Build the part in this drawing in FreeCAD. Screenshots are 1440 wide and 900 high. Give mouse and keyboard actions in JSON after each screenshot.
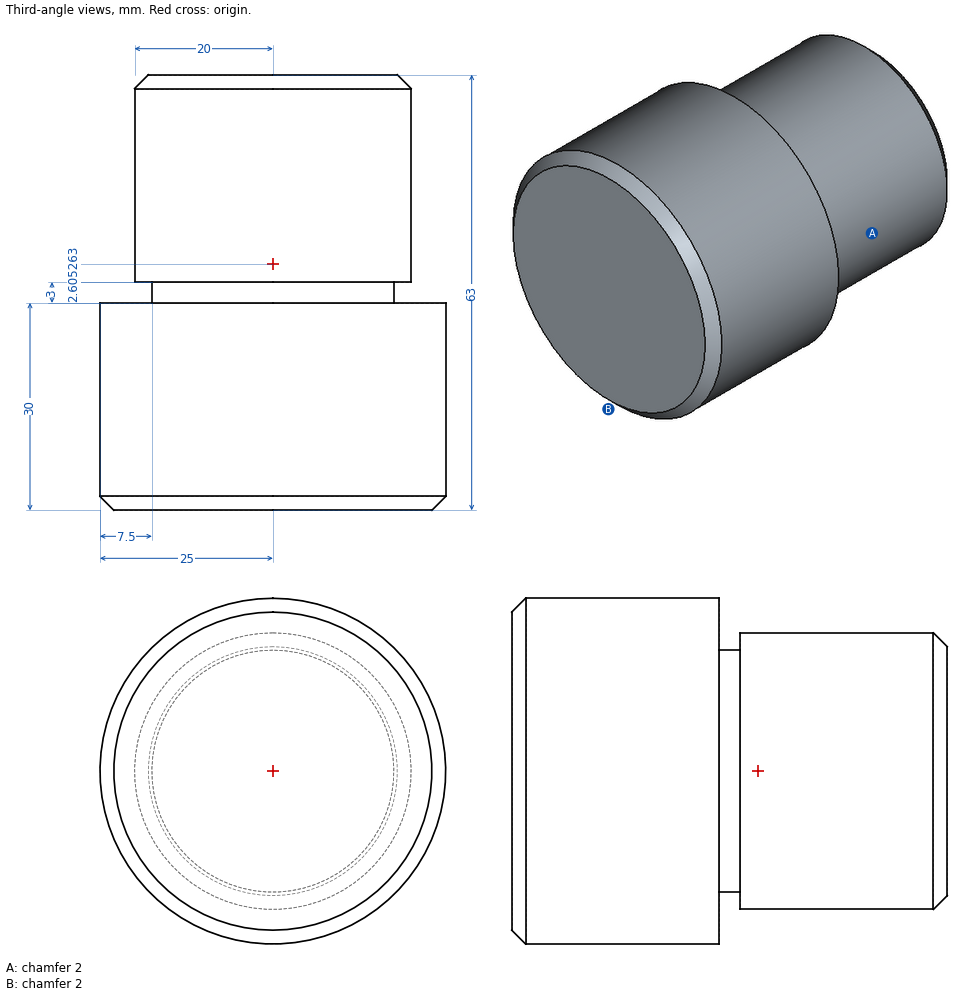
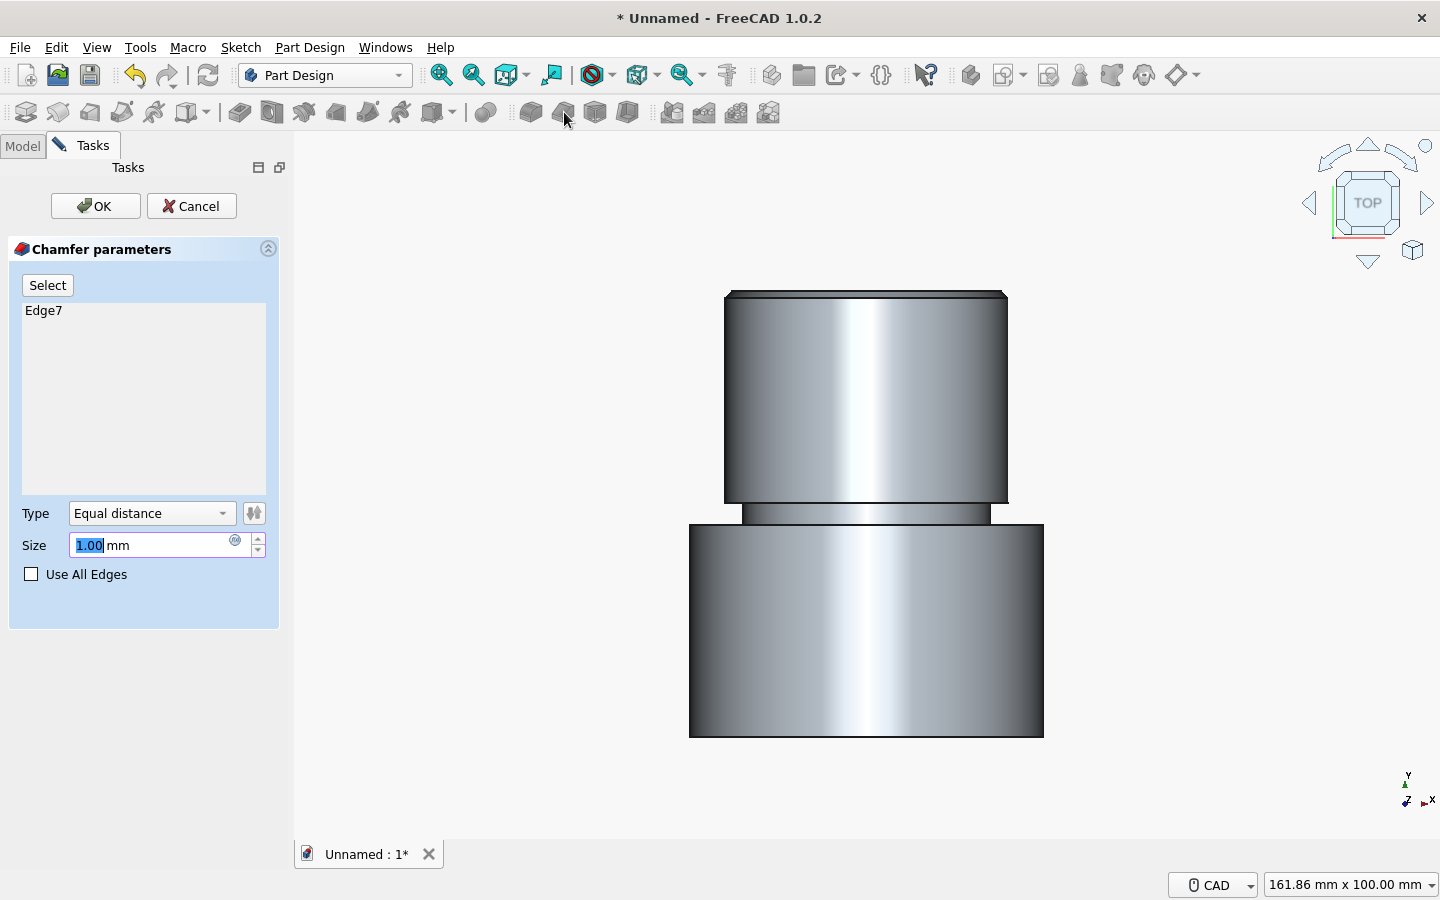
{"action": "type", "text": "2"}
{"action": "key", "text": "Tab"}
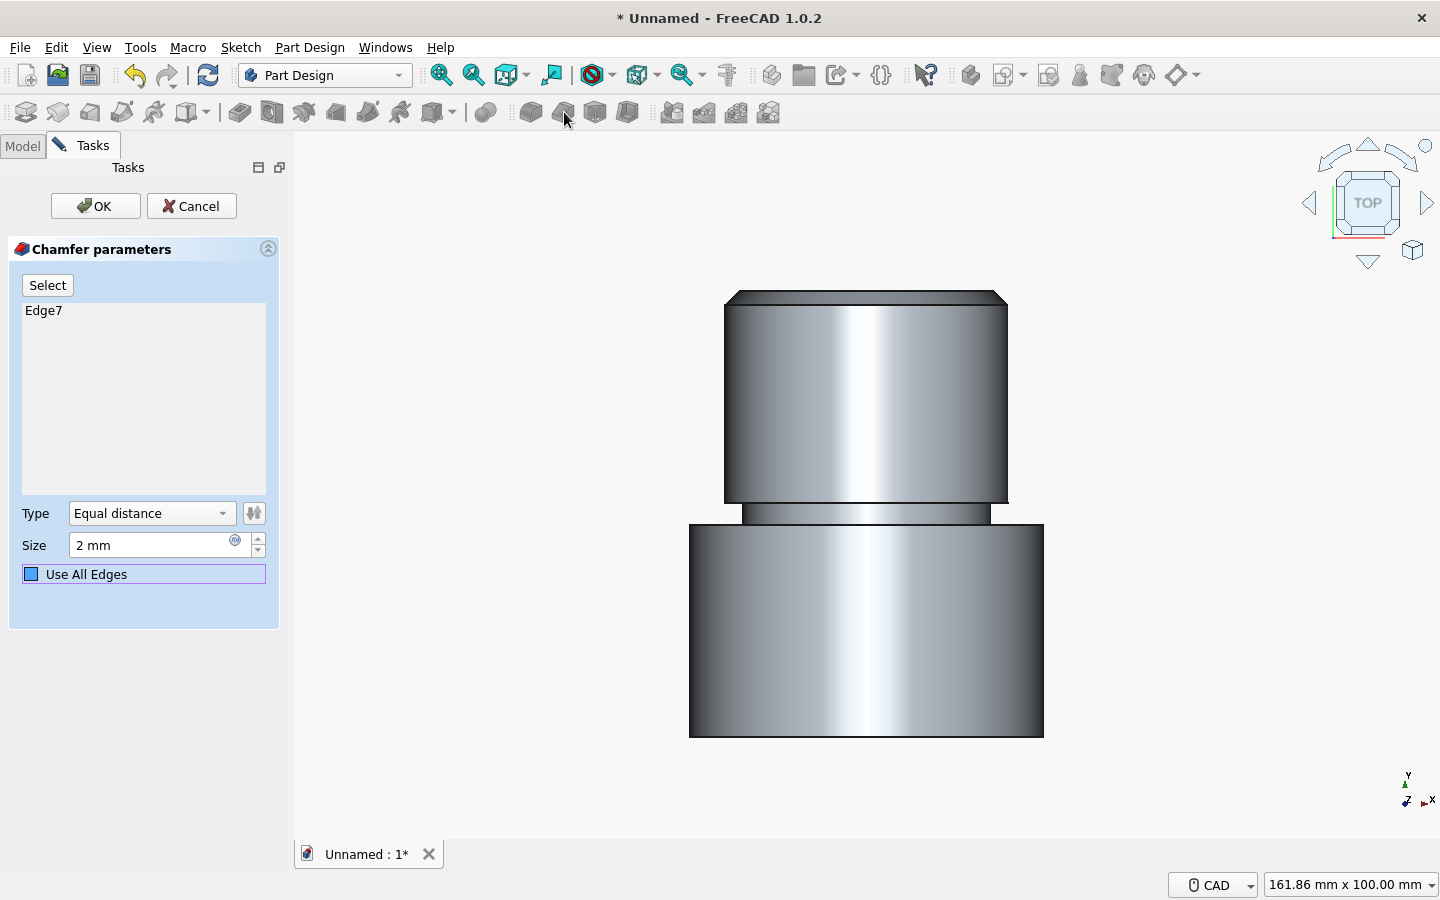
{"action": "left_click", "coordinate": [96, 206]}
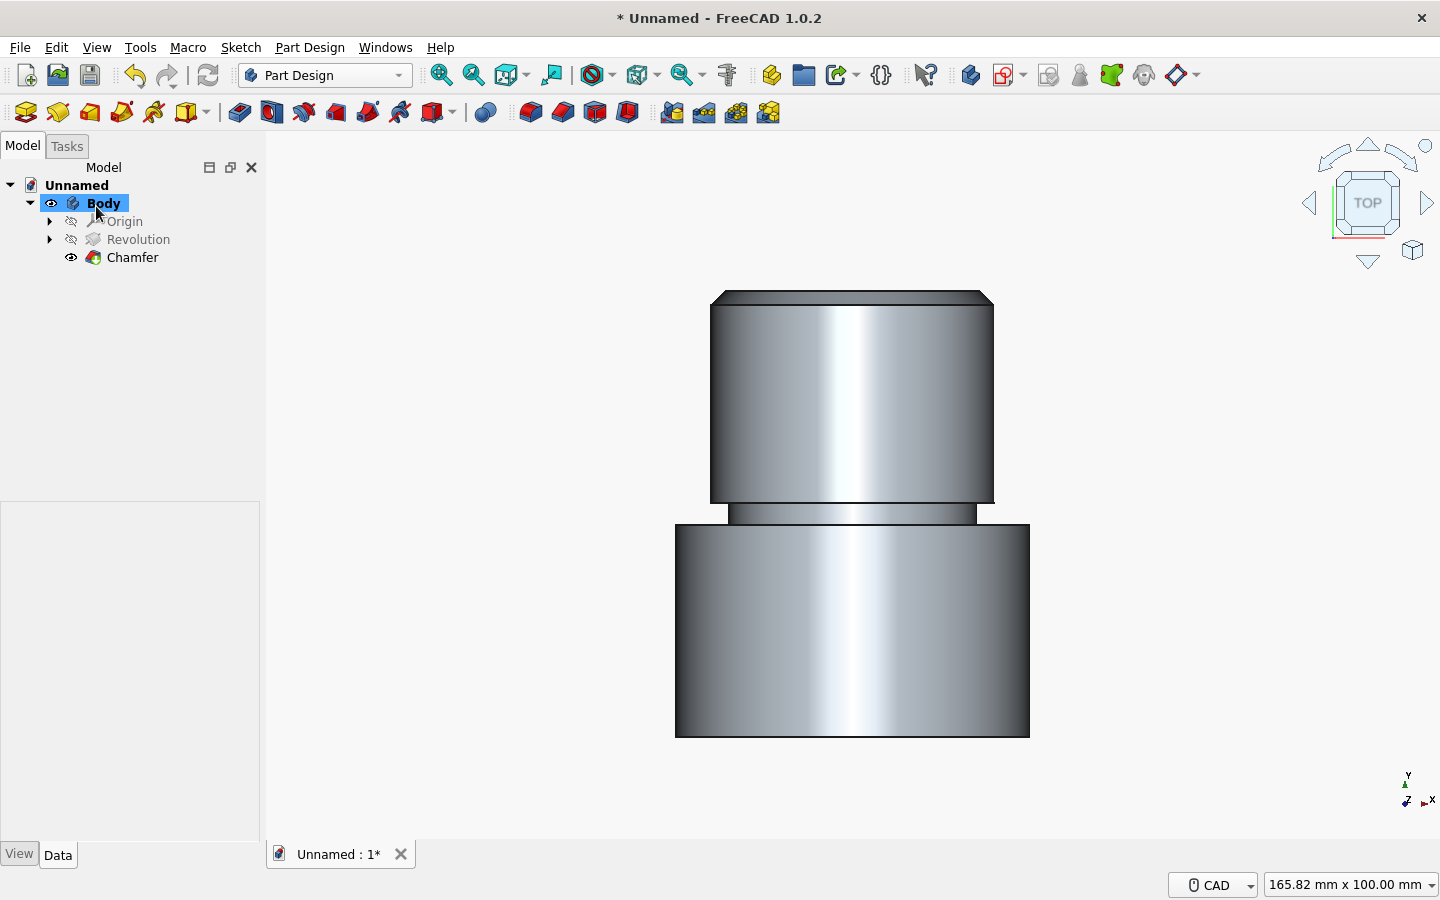
{"action": "left_click", "coordinate": [996, 736]}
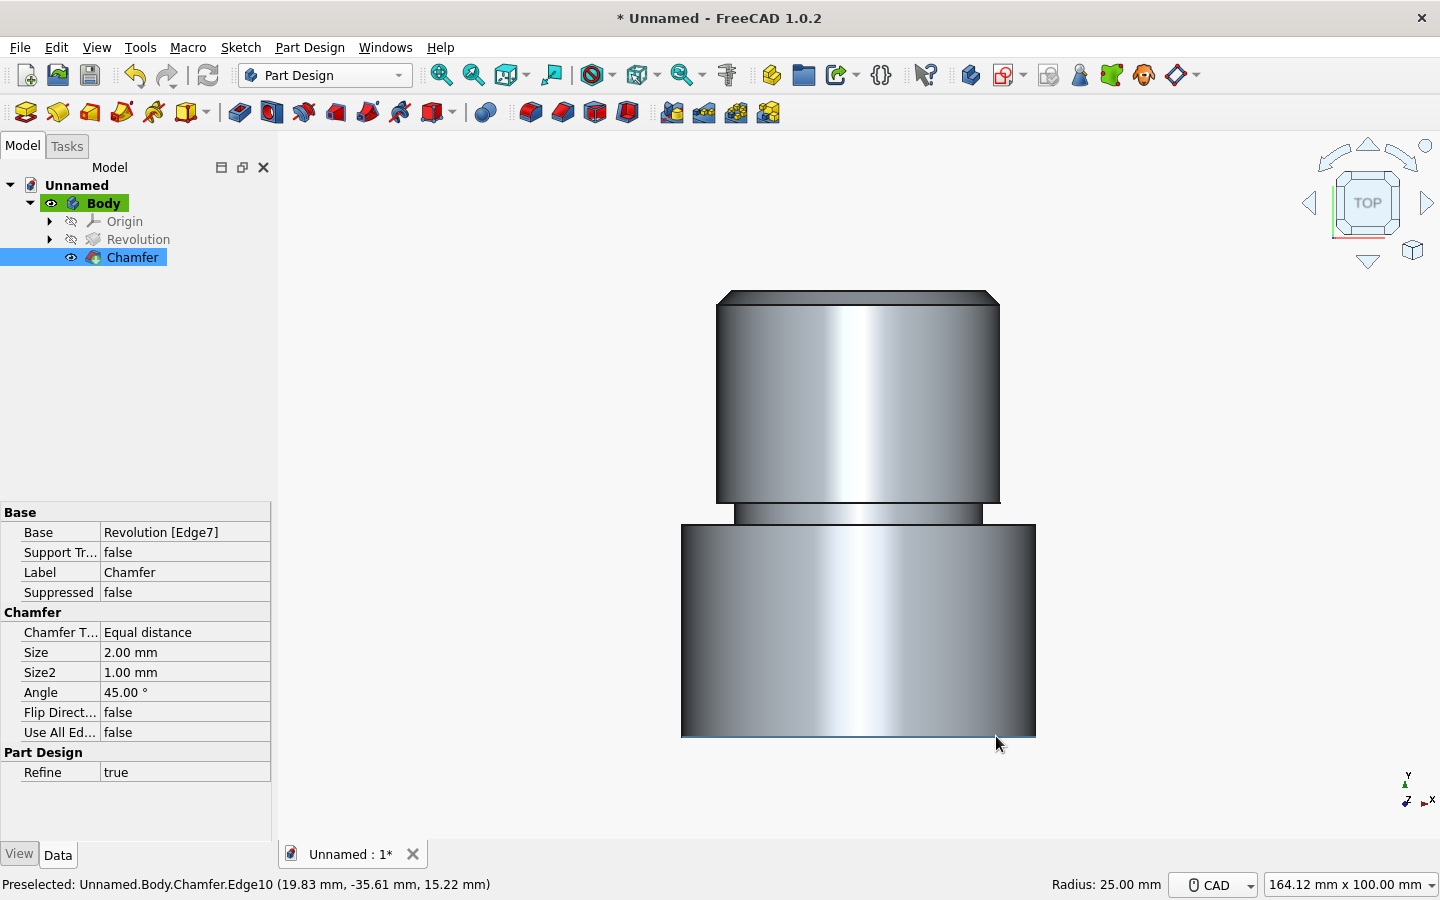
{"action": "left_click", "coordinate": [564, 112]}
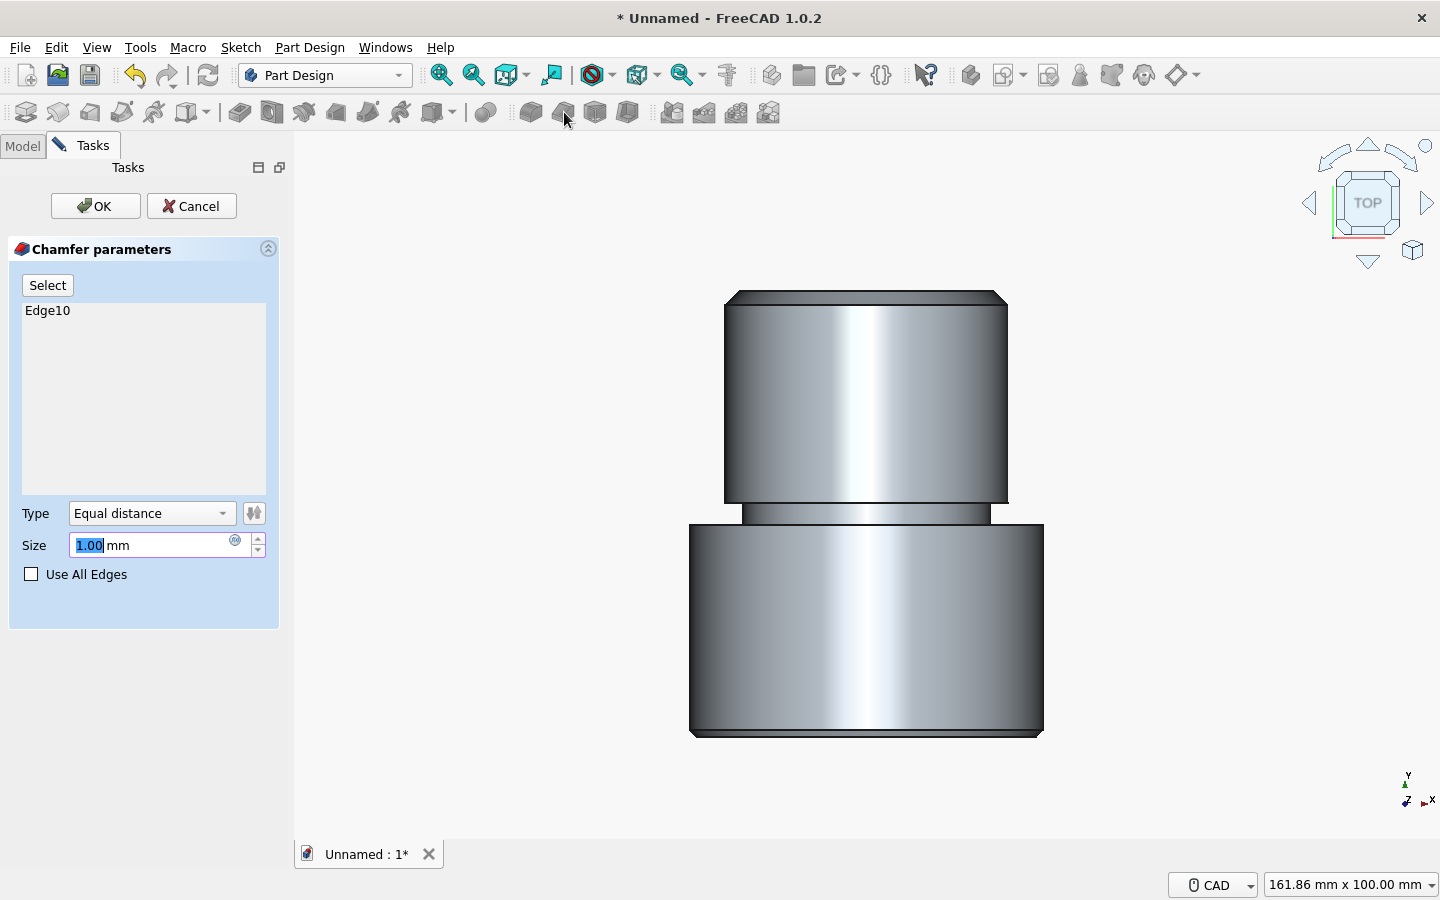
{"action": "type", "text": "2"}
{"action": "key", "text": "Tab"}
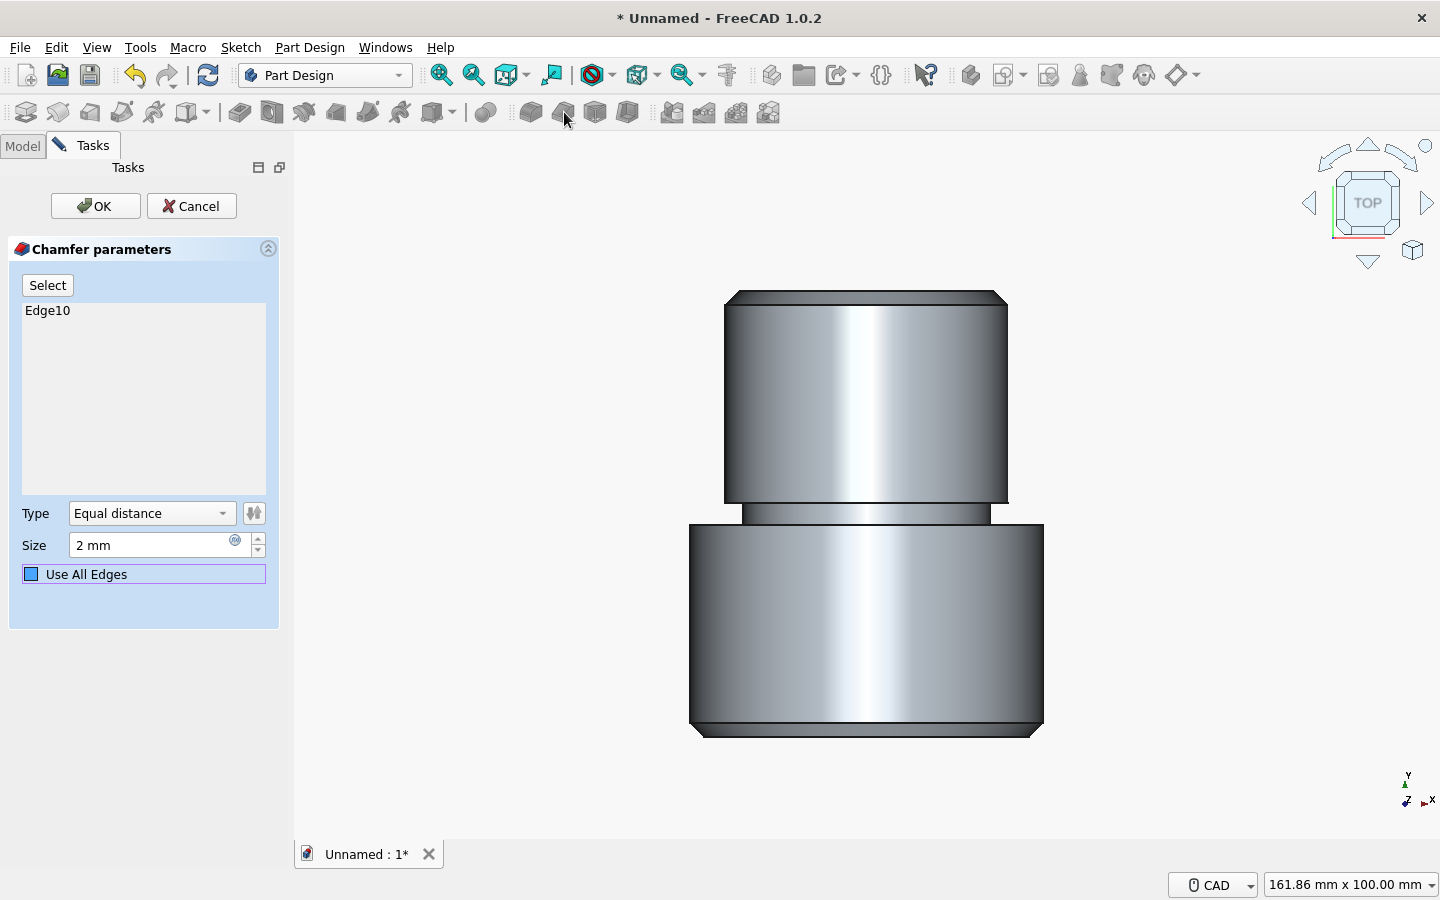
{"action": "left_click", "coordinate": [96, 206]}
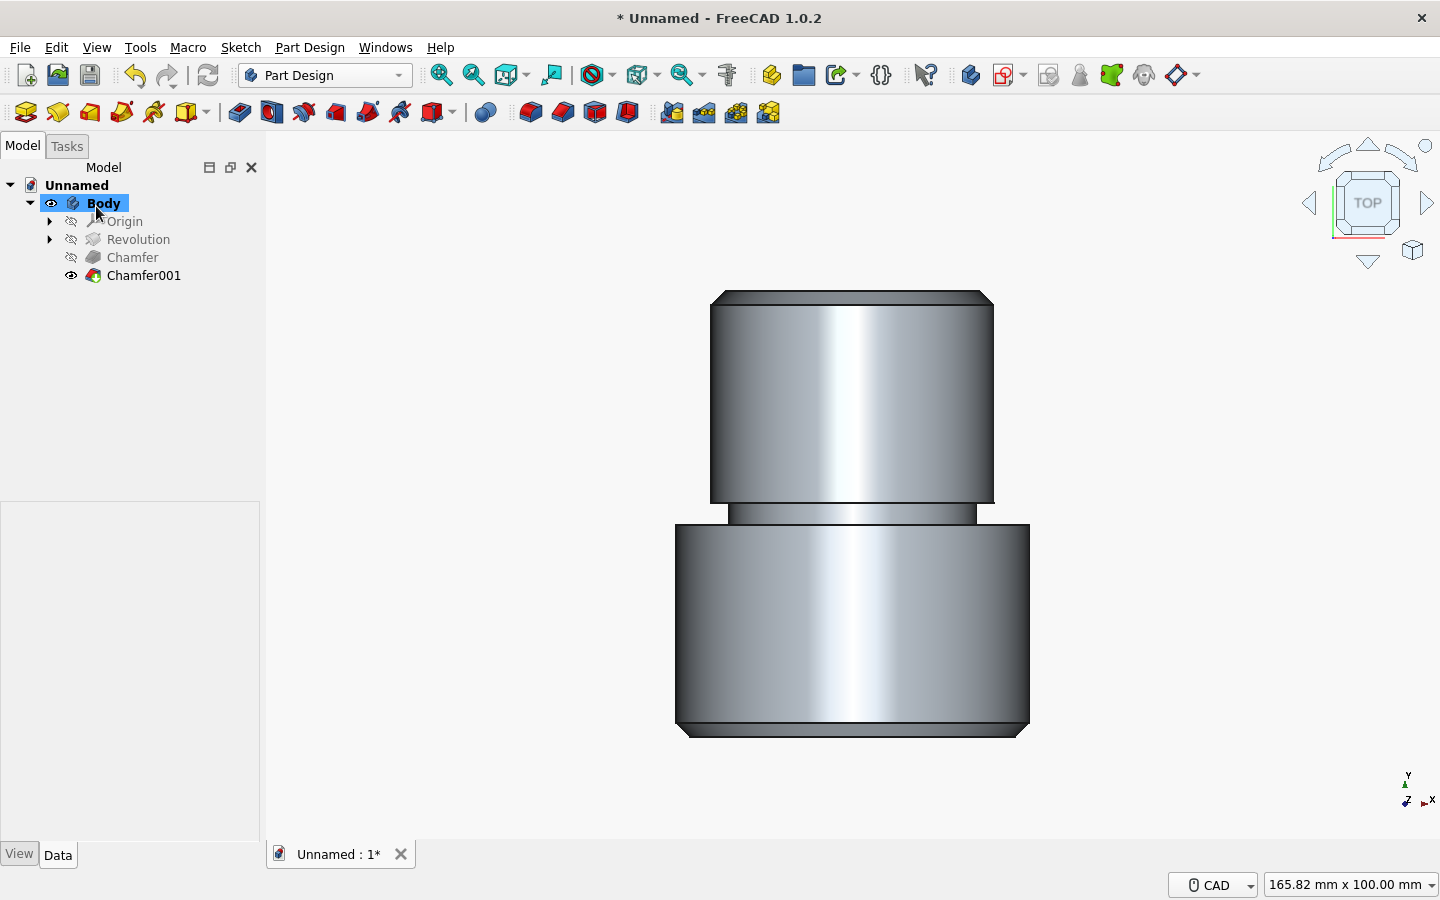
{"action": "key", "text": "0"}